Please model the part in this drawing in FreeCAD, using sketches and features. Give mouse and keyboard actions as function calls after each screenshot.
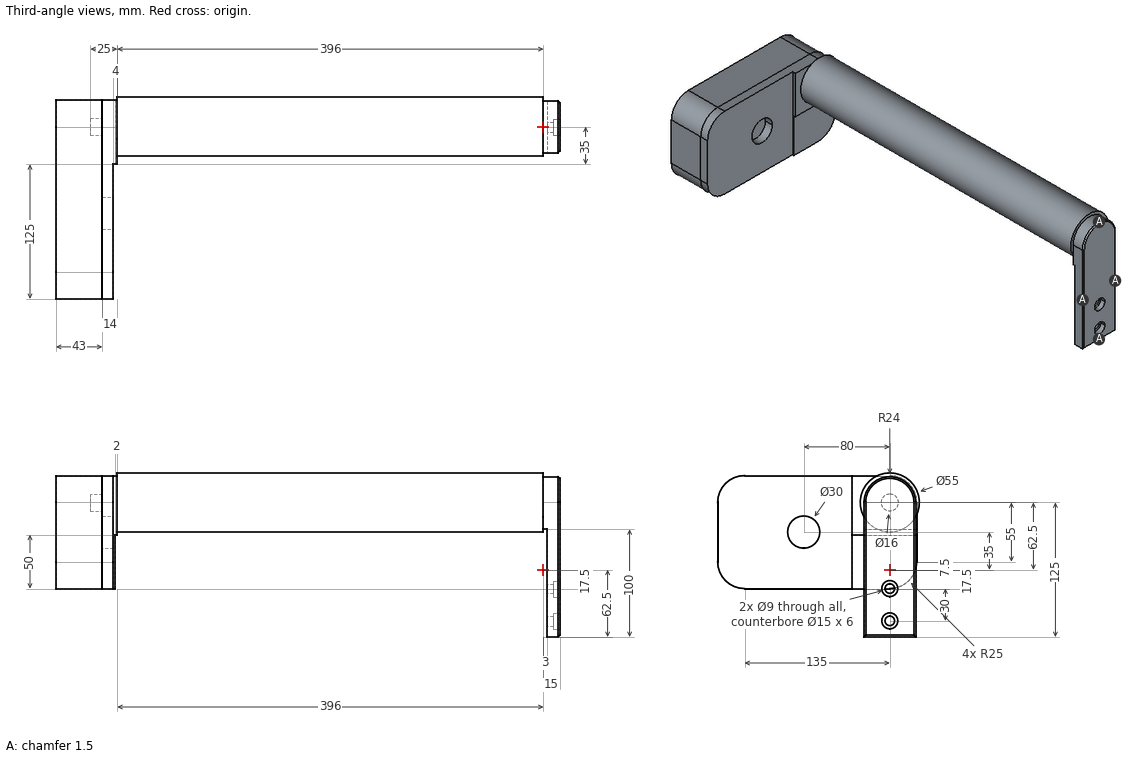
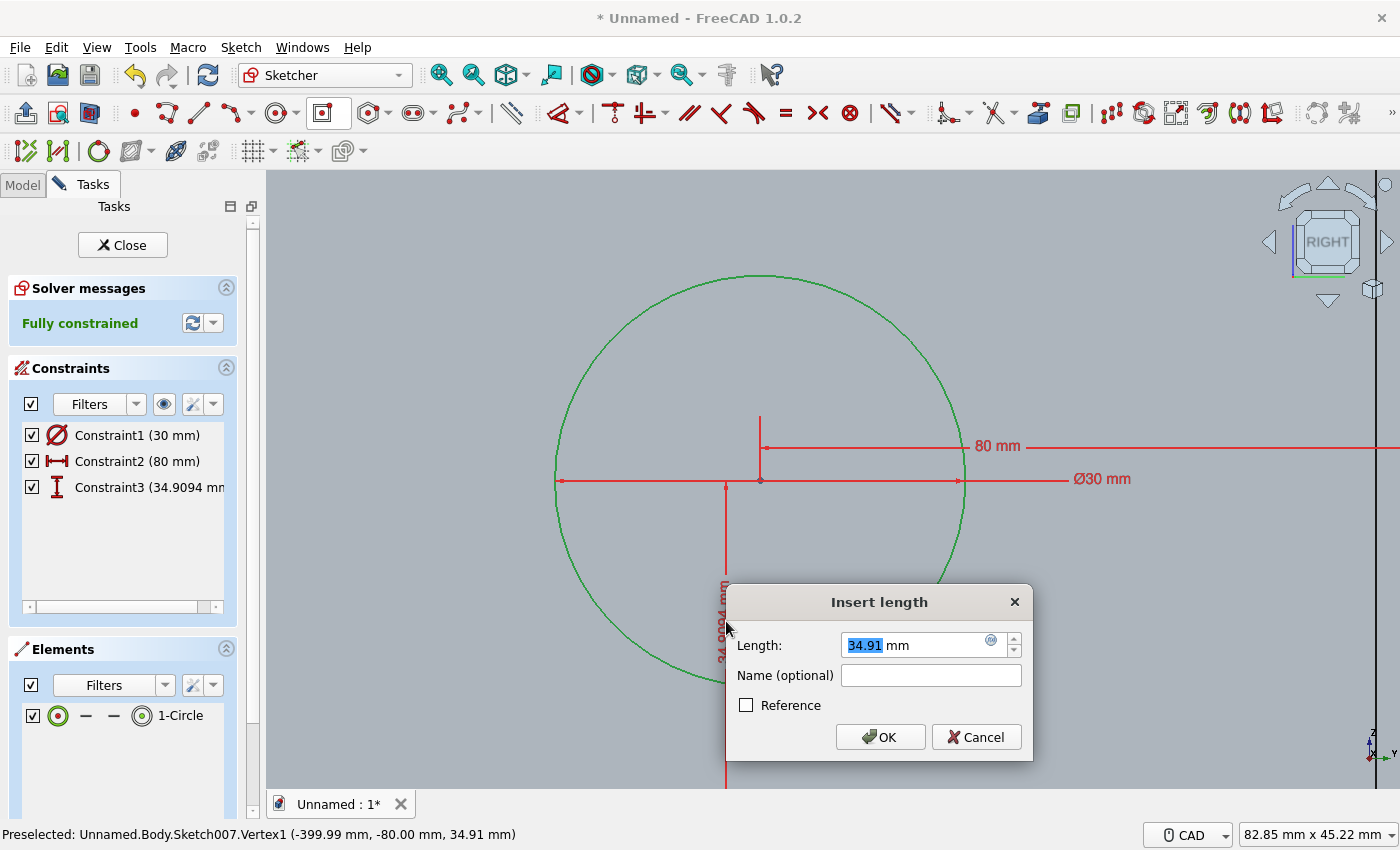
text(35)
key(Return)
key(Escape)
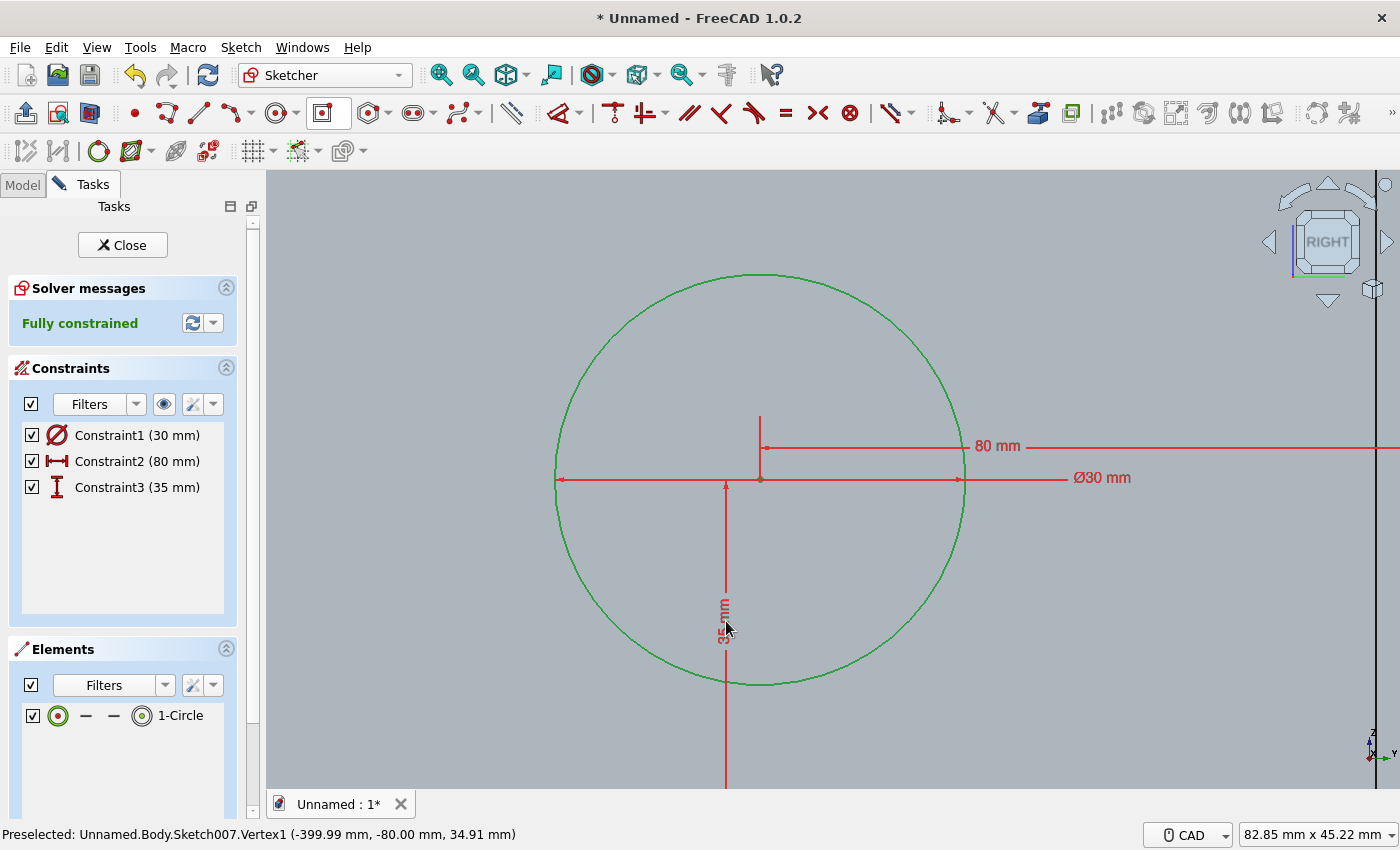
click(123, 245)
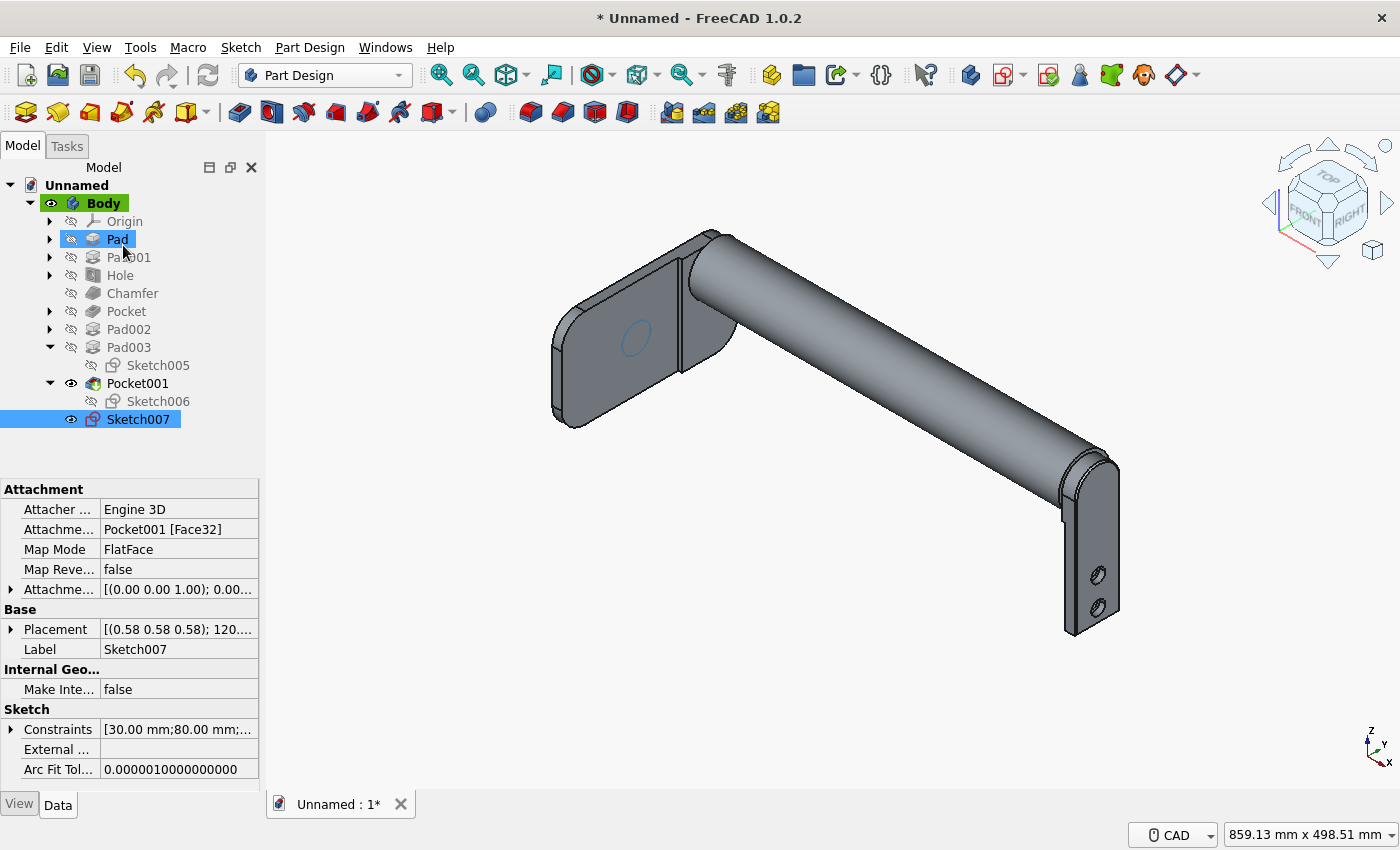
click(240, 112)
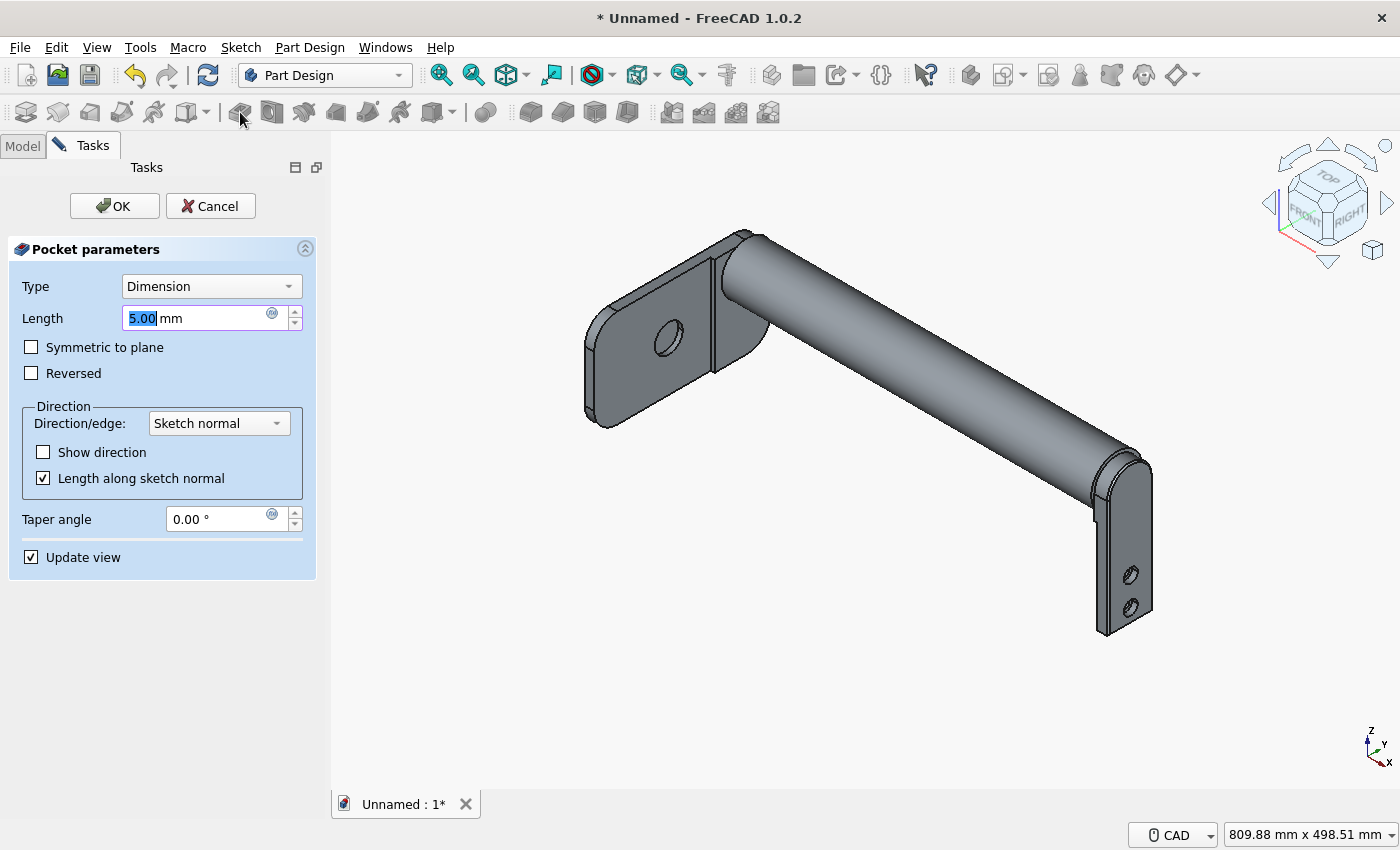
click(212, 286)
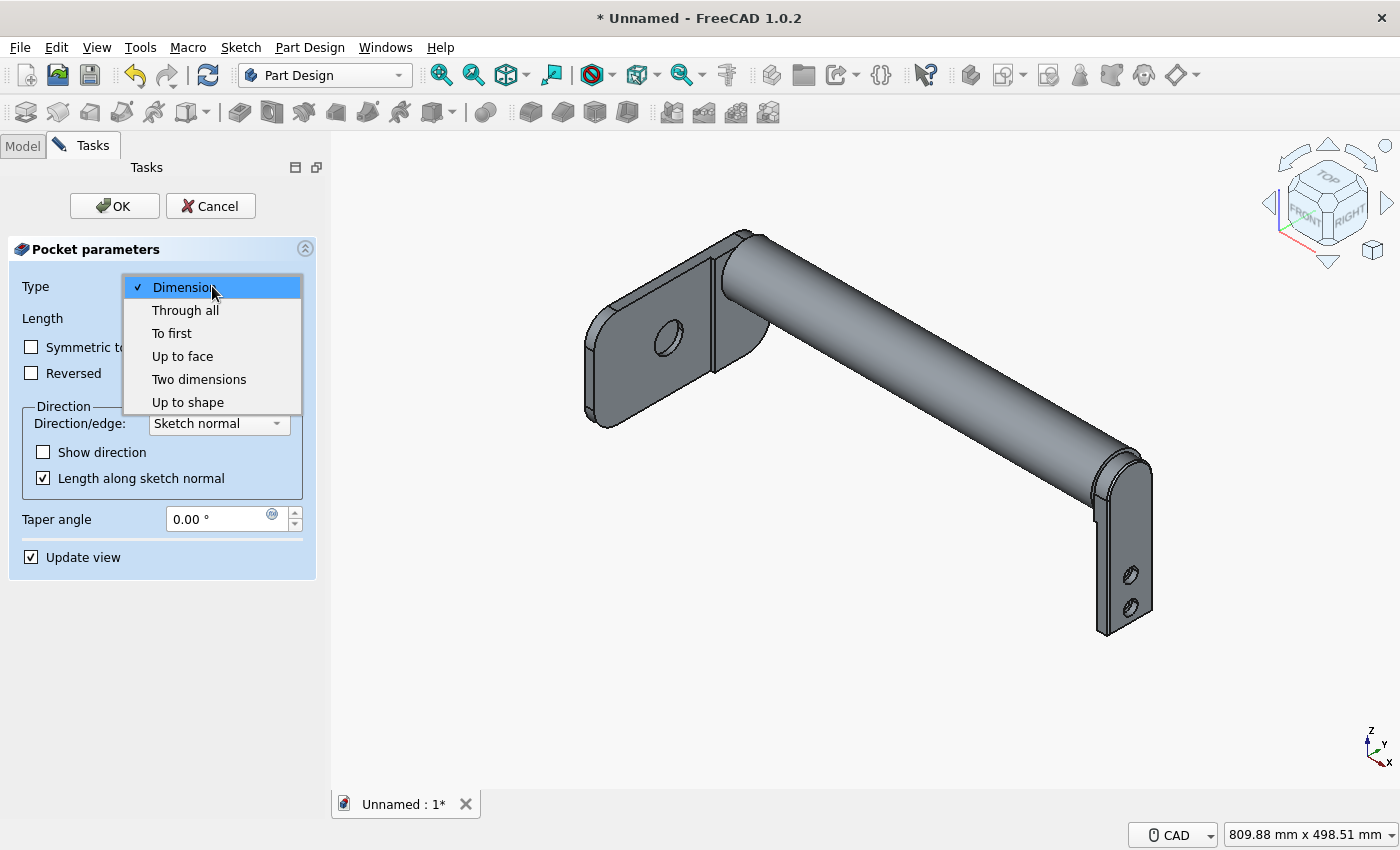
click(212, 310)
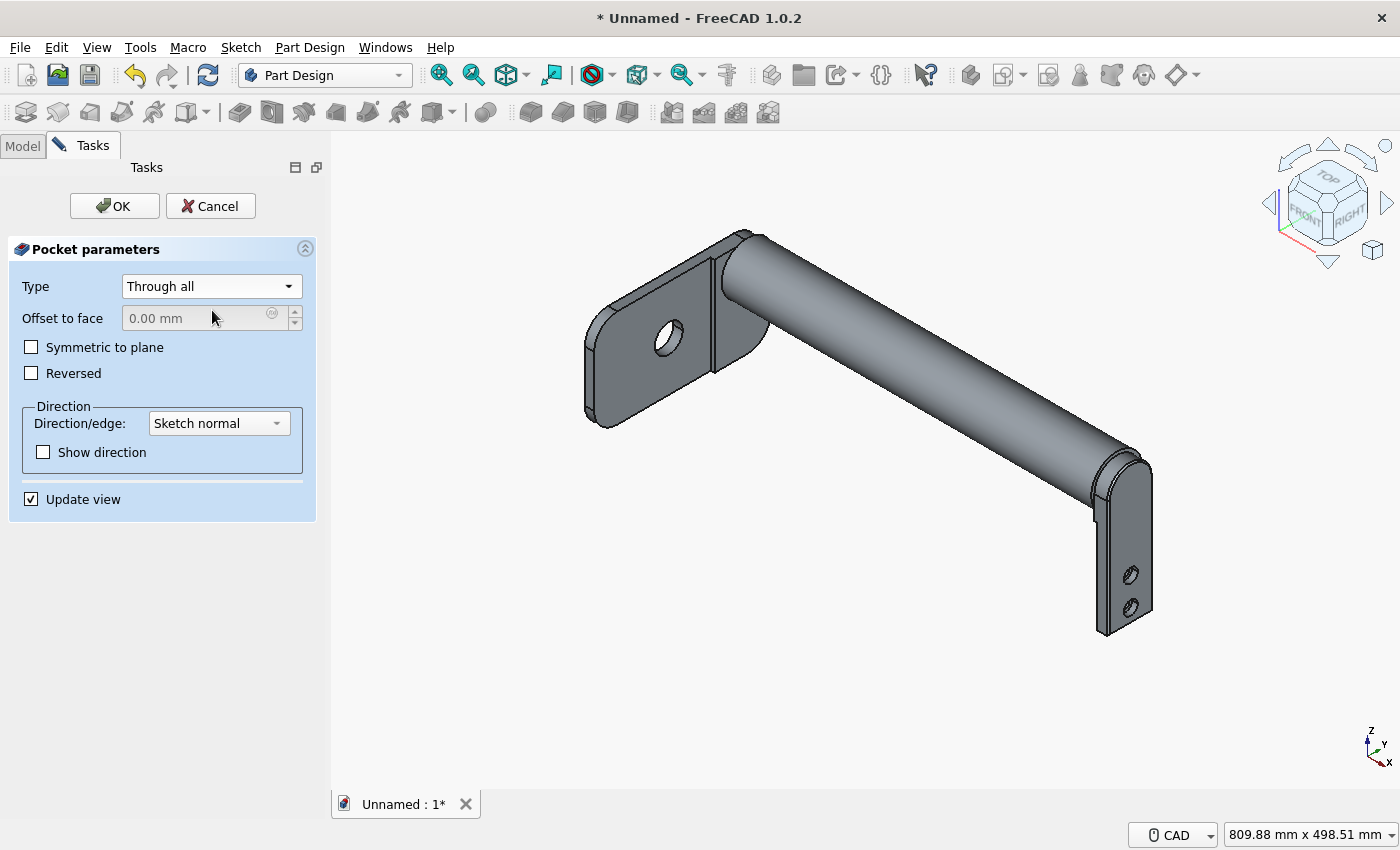
click(115, 206)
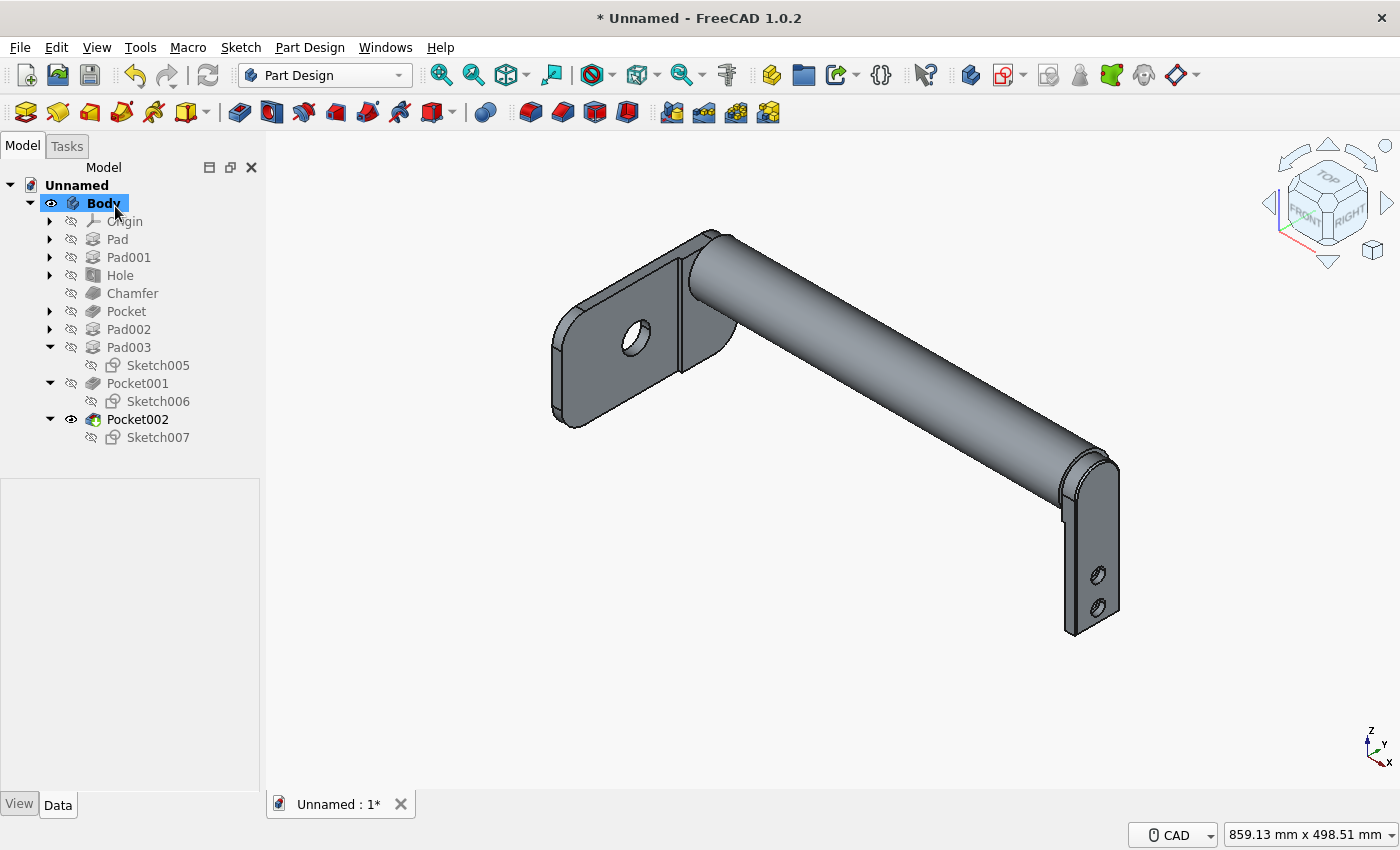
key(4)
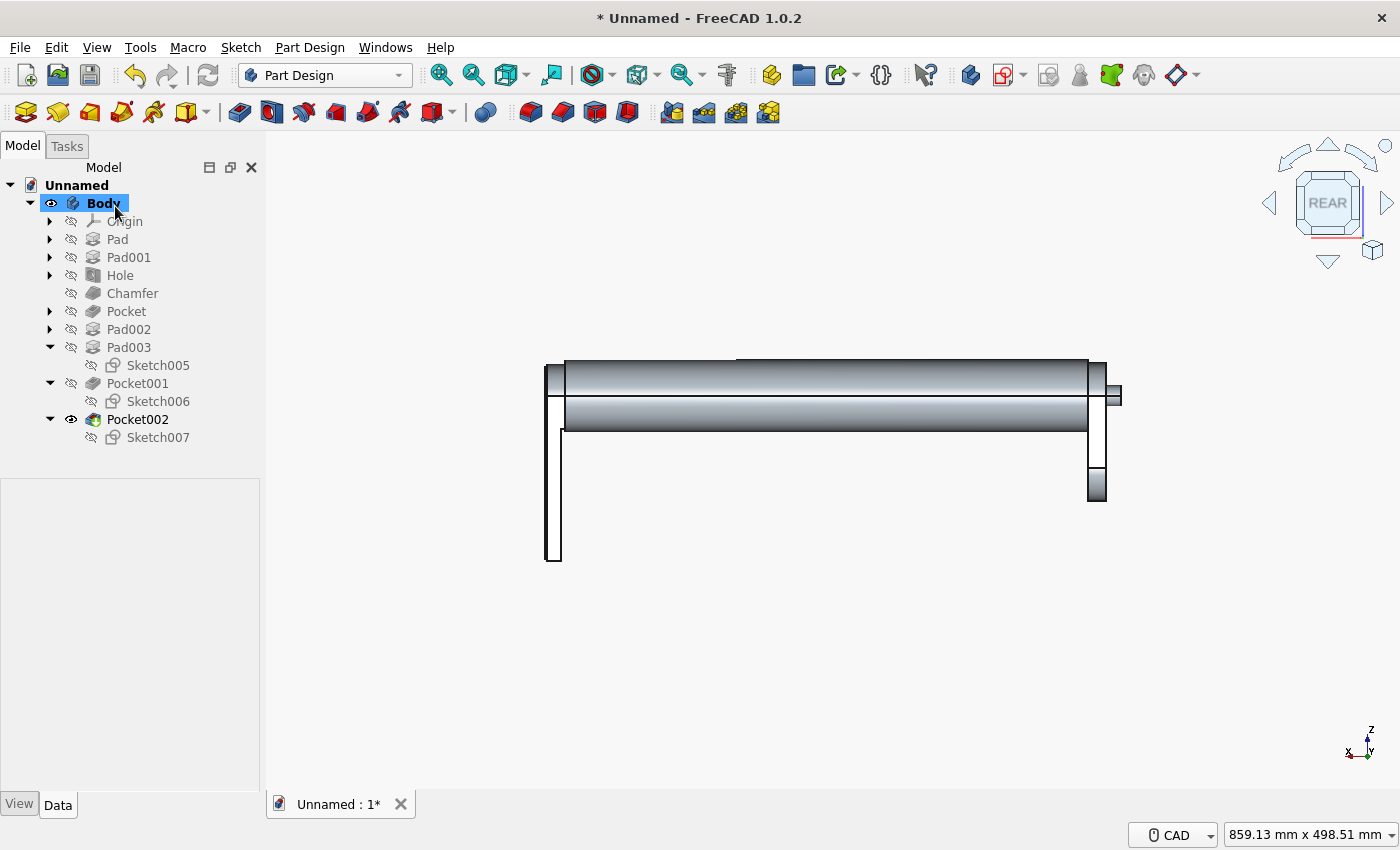
click(1097, 441)